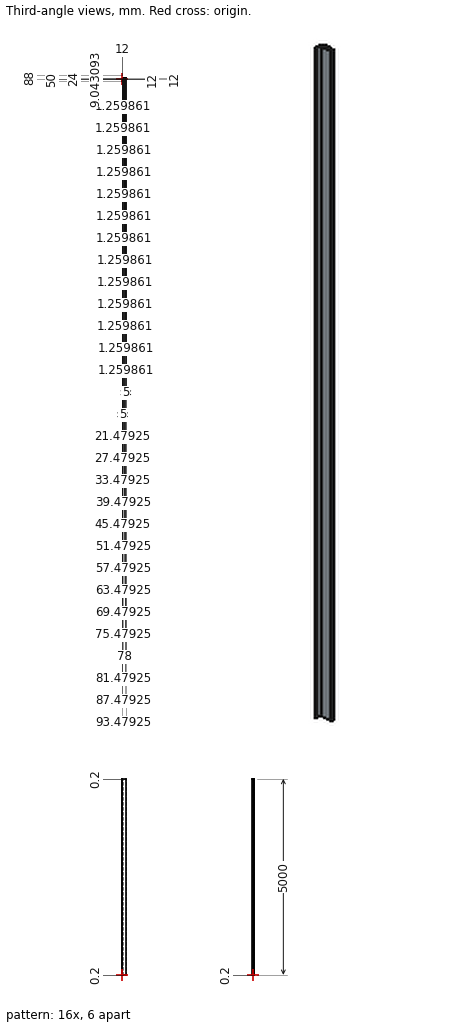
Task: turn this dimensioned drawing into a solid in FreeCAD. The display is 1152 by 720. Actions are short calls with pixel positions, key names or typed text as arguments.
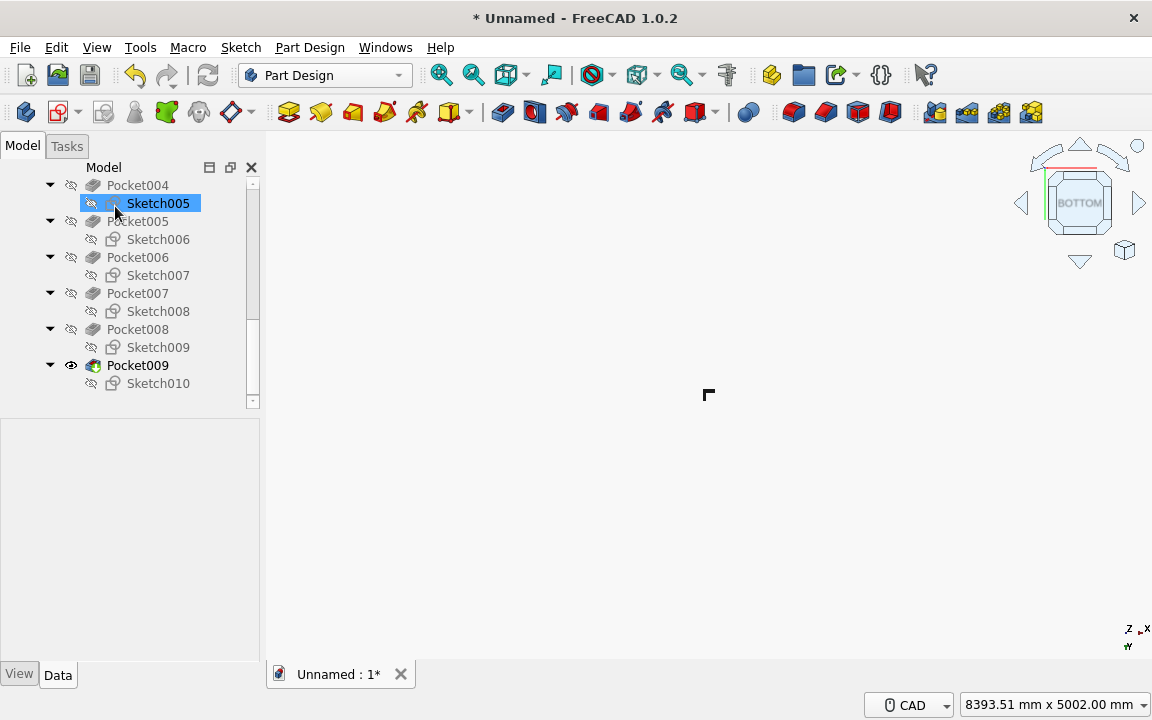
key(v)
key(f)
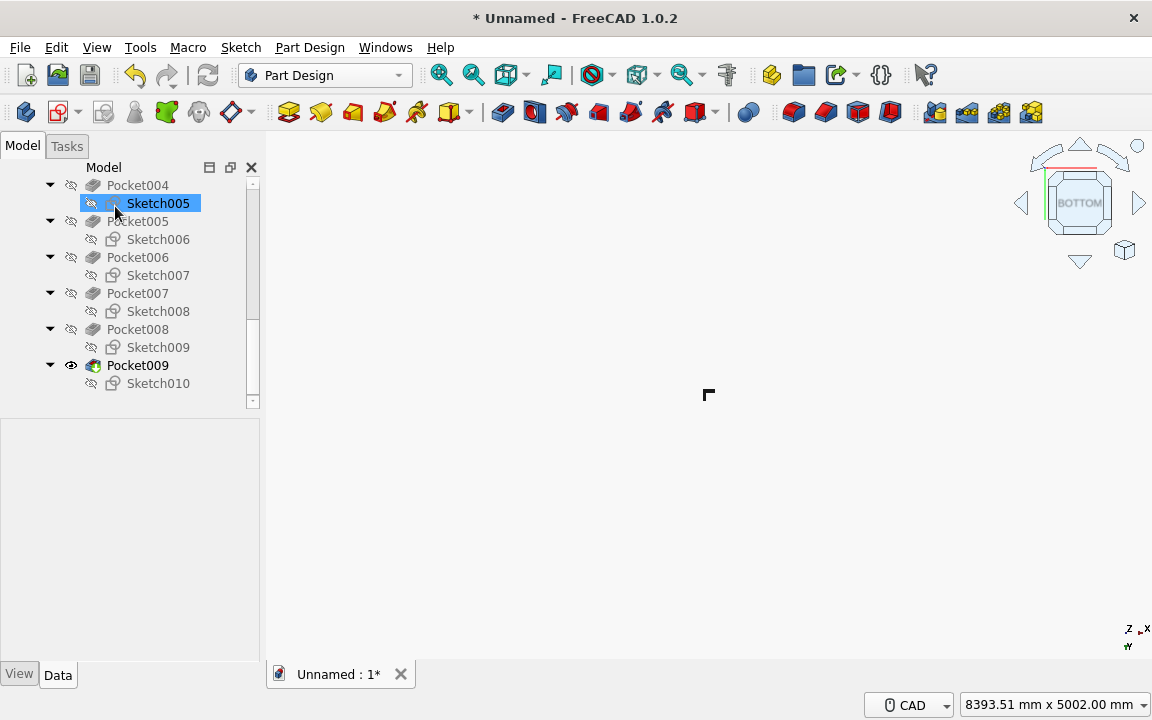
scroll(712, 389, up, 14)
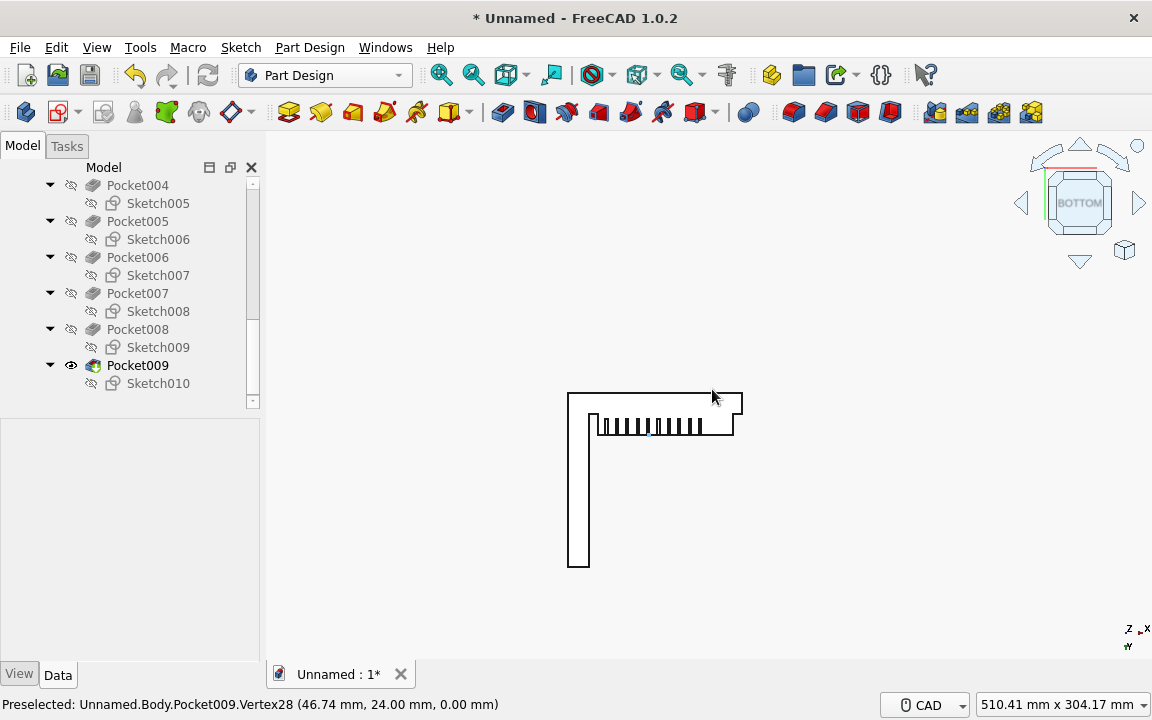
click(704, 405)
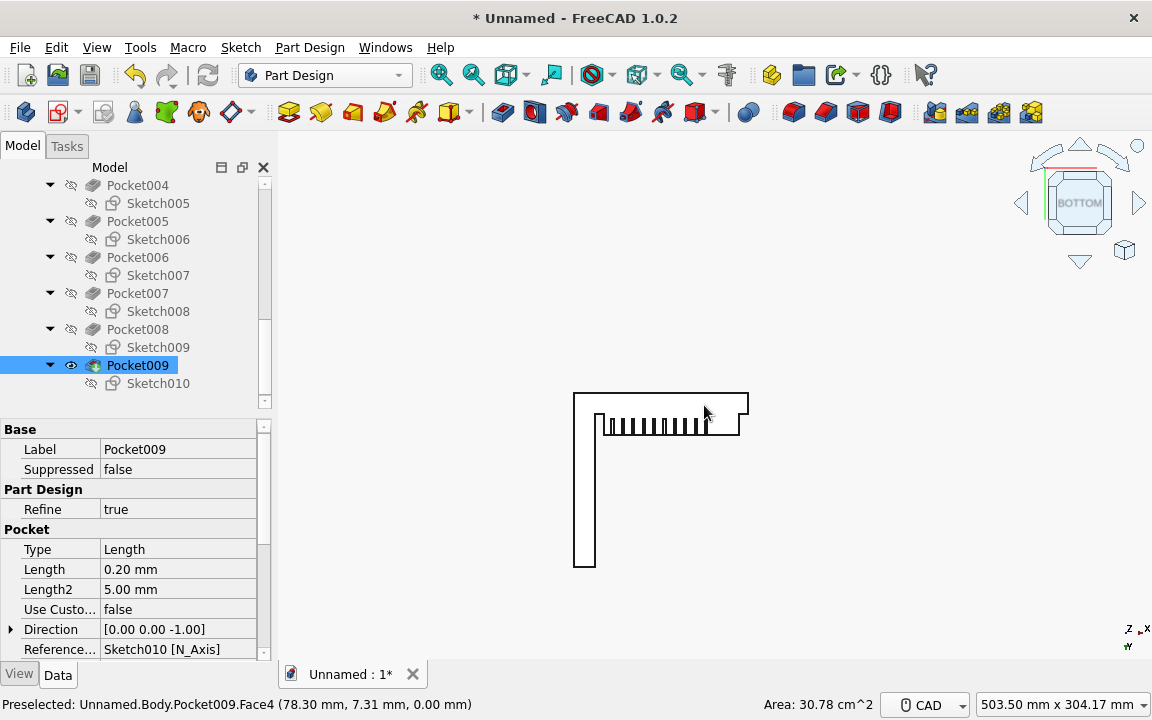
click(58, 112)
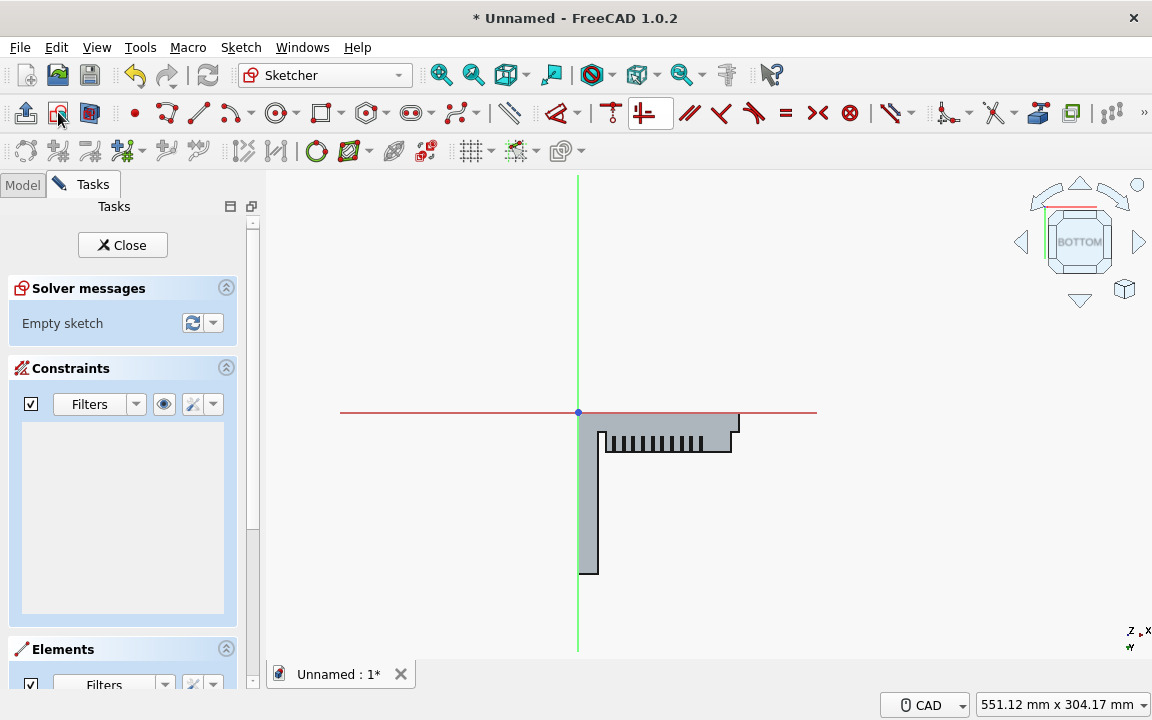
scroll(714, 446, up, 15)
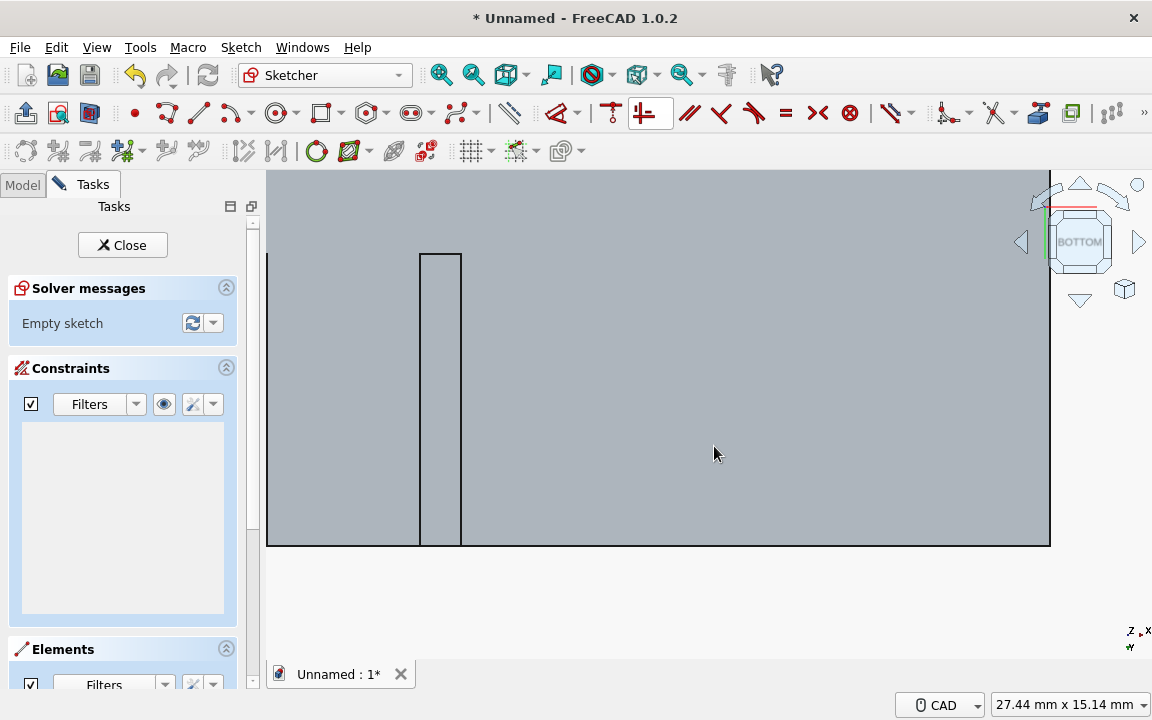
click(322, 114)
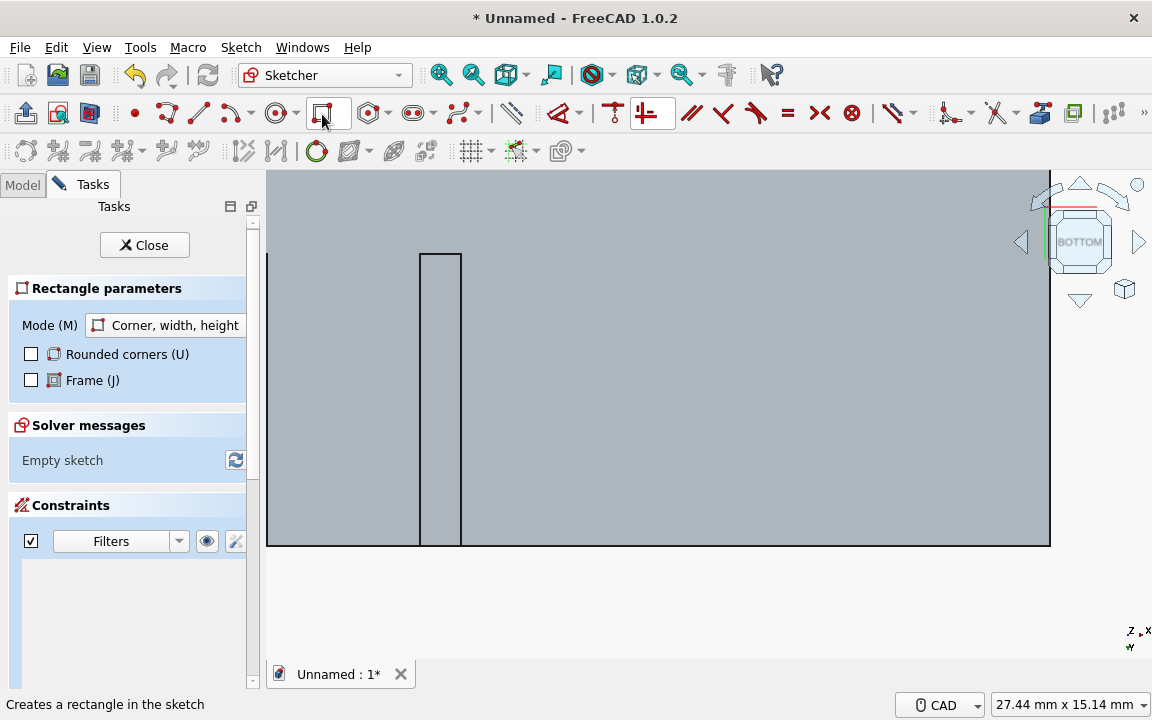
click(614, 254)
click(654, 546)
key(Escape)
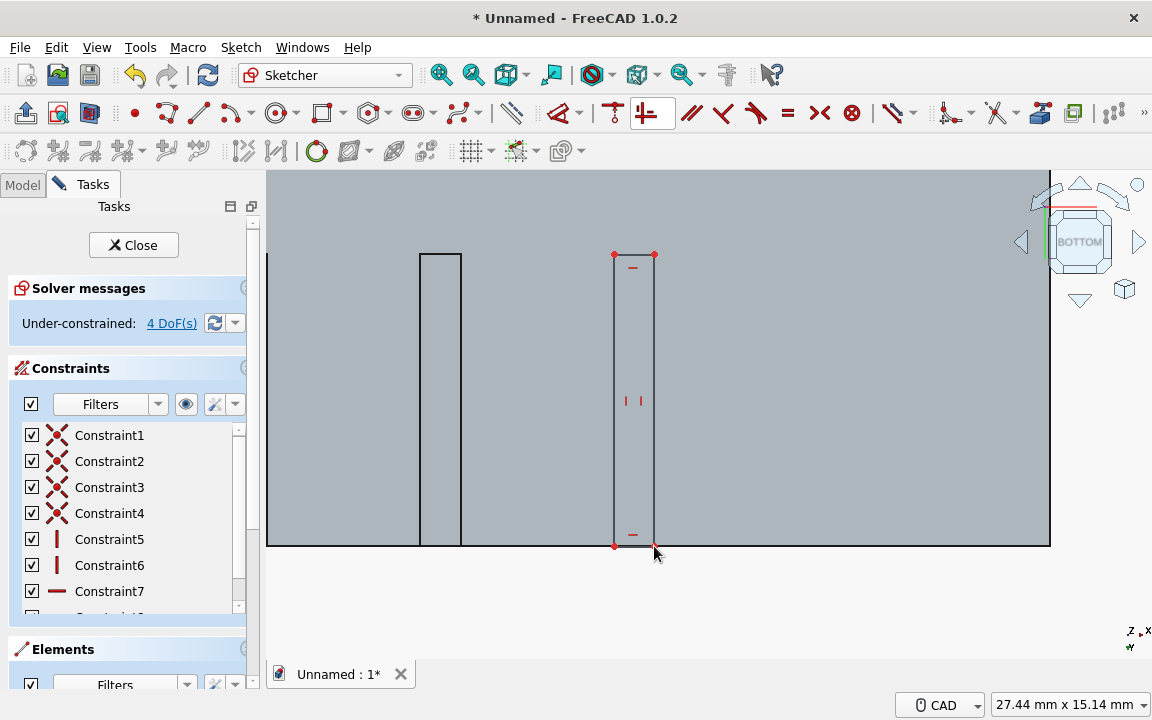
click(558, 114)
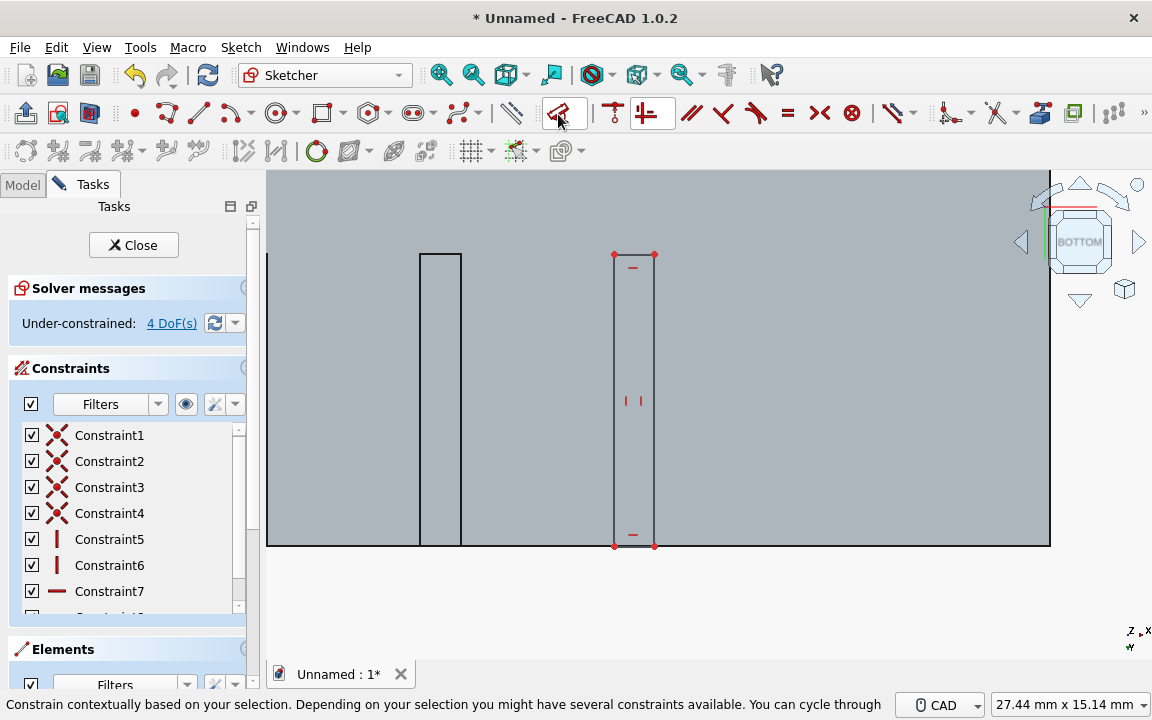
click(614, 547)
click(672, 373)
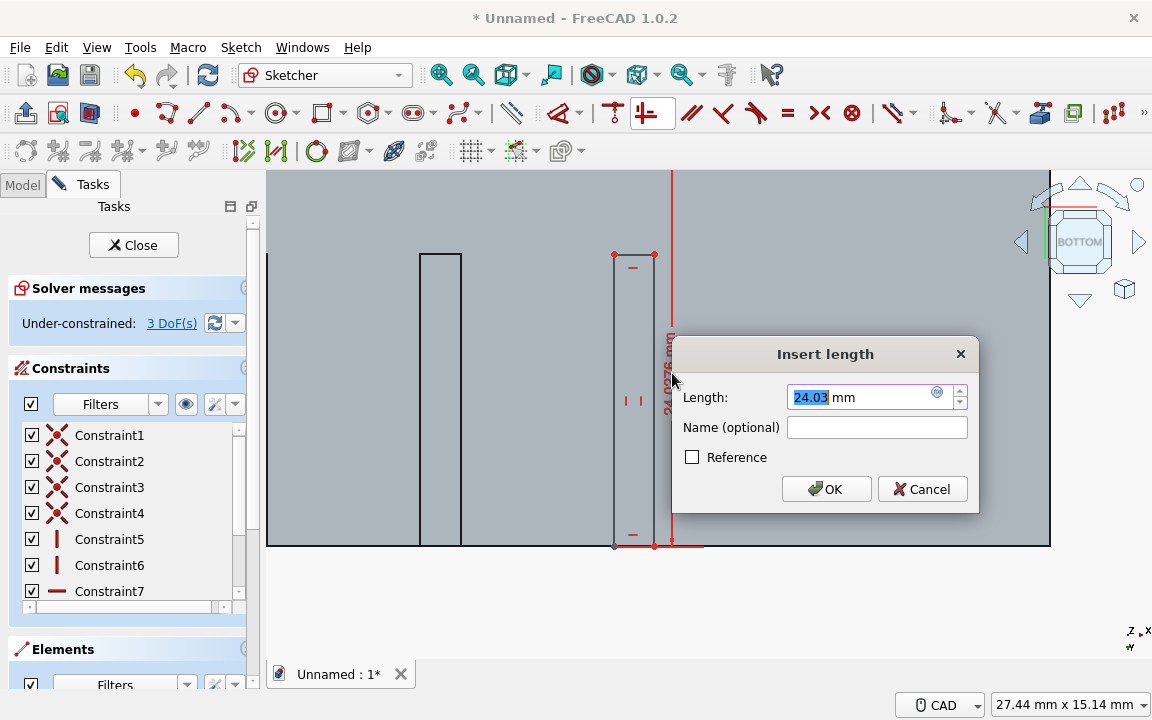
text(24)
key(Return)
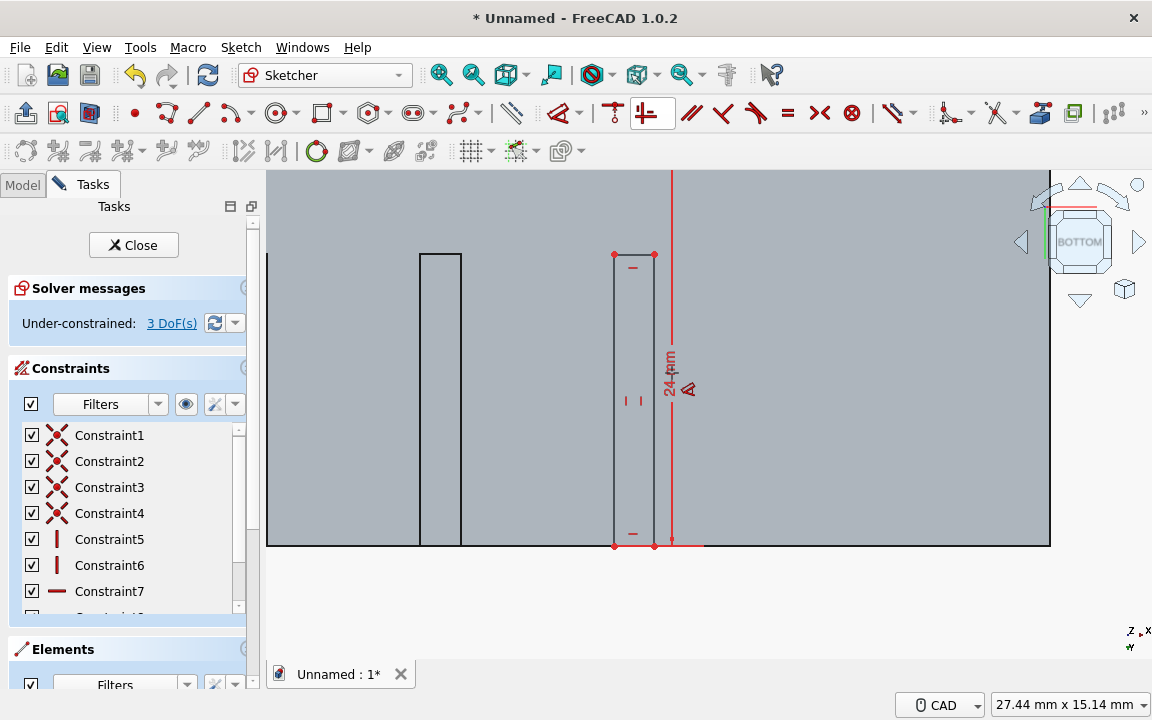
click(614, 342)
click(580, 401)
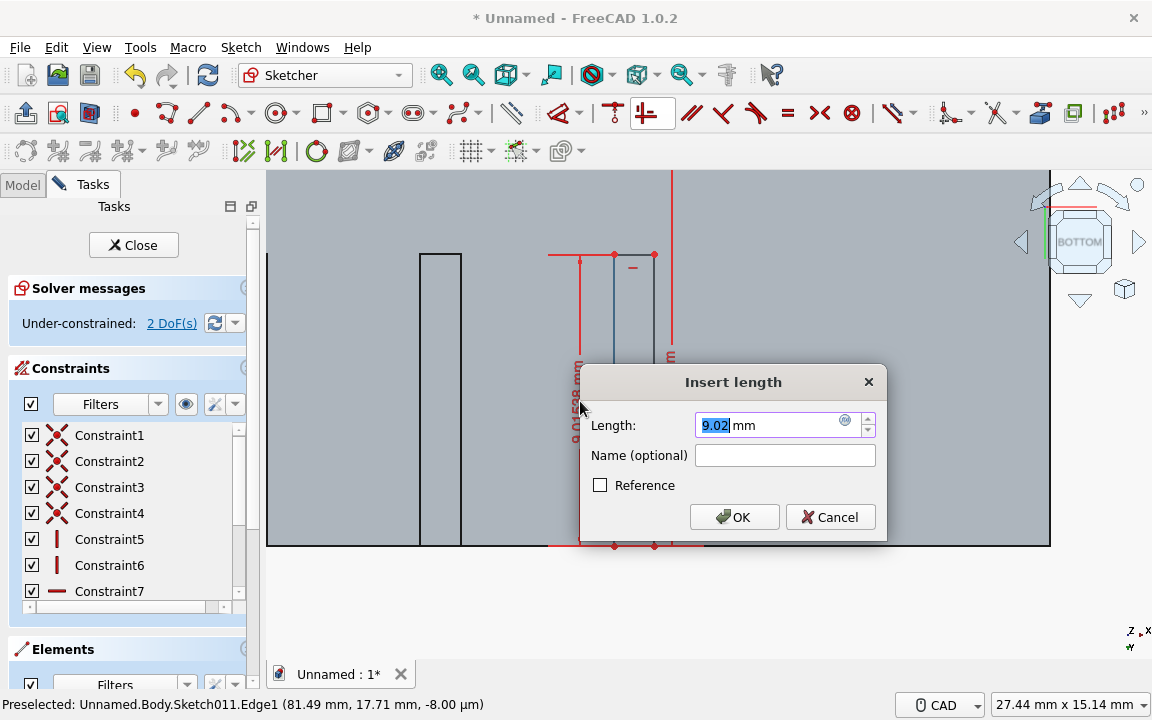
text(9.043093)
key(Return)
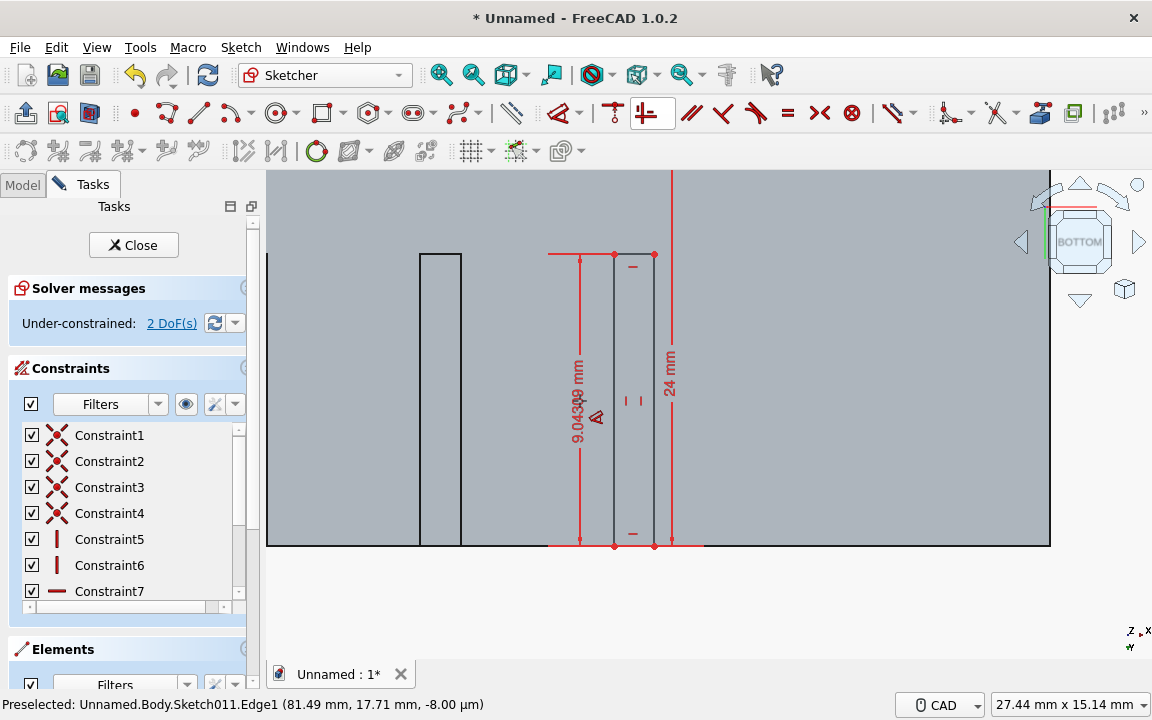
click(626, 546)
click(634, 580)